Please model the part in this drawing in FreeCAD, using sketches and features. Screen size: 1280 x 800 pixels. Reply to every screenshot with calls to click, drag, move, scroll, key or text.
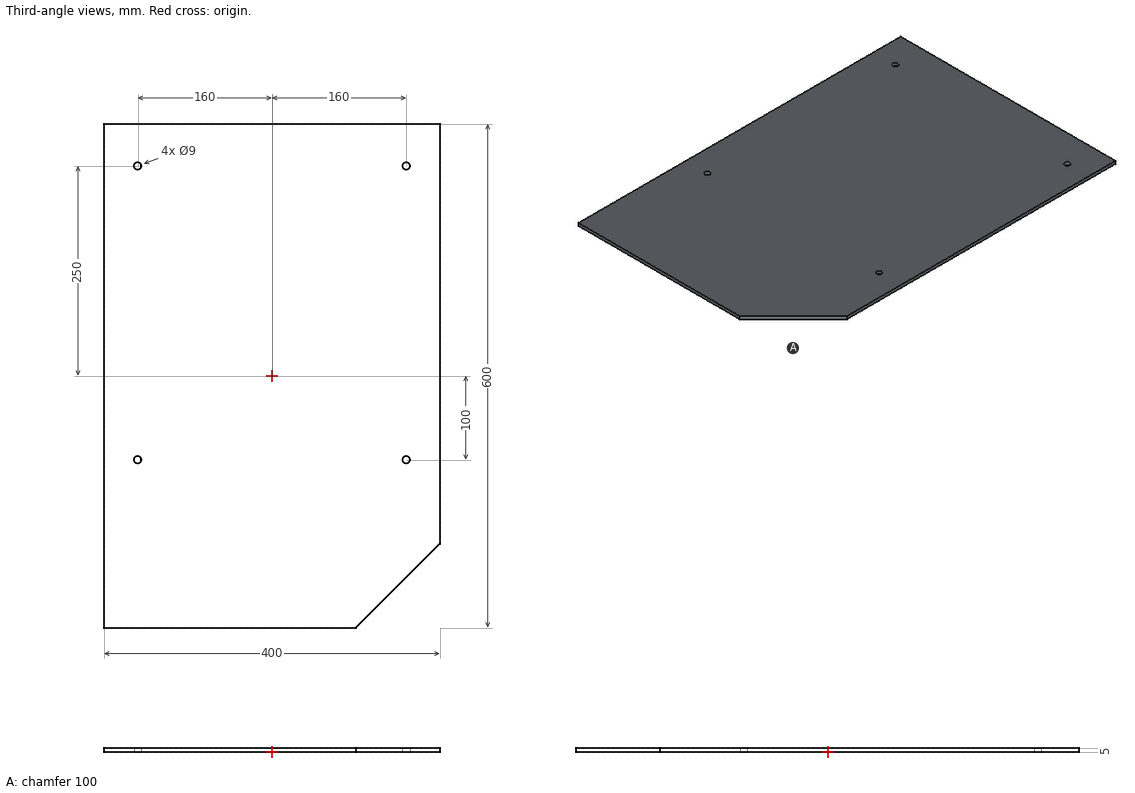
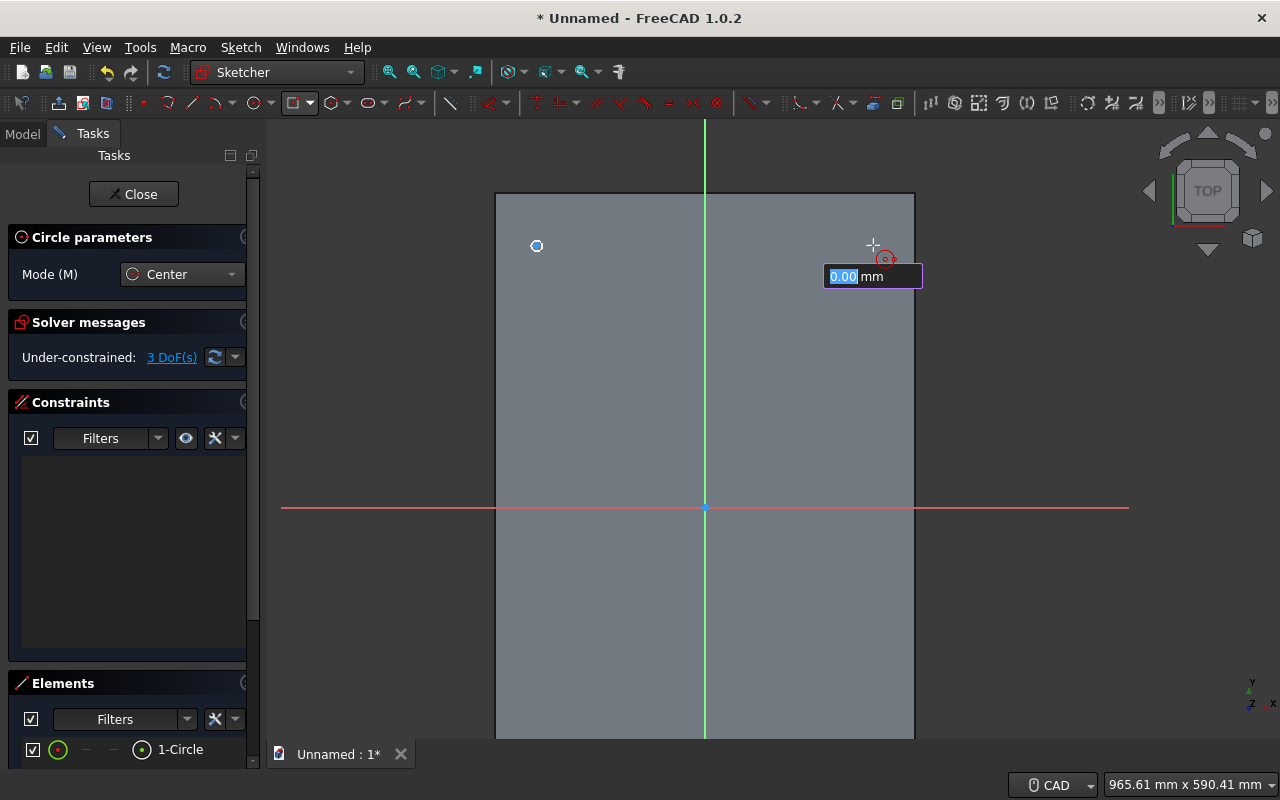
scroll(877, 242, up, 7)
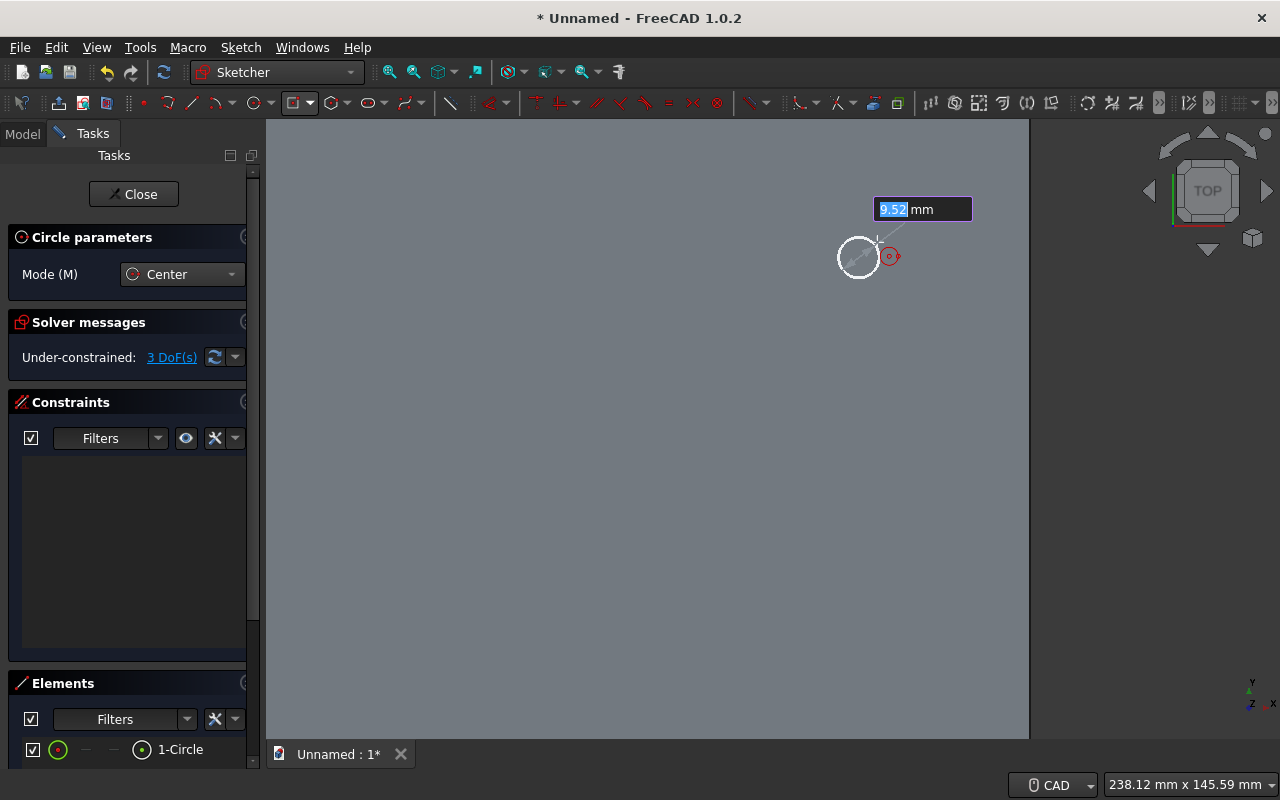
click(873, 241)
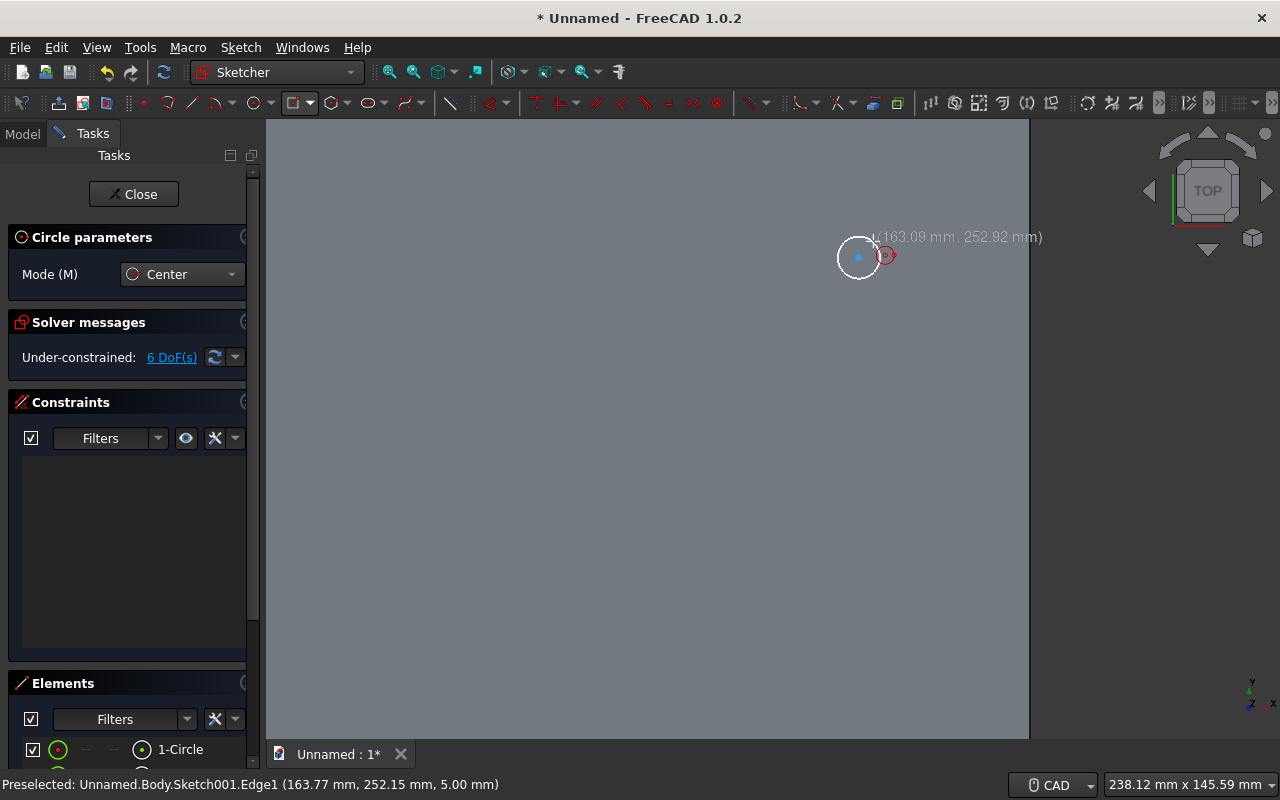
scroll(877, 242, down, 7)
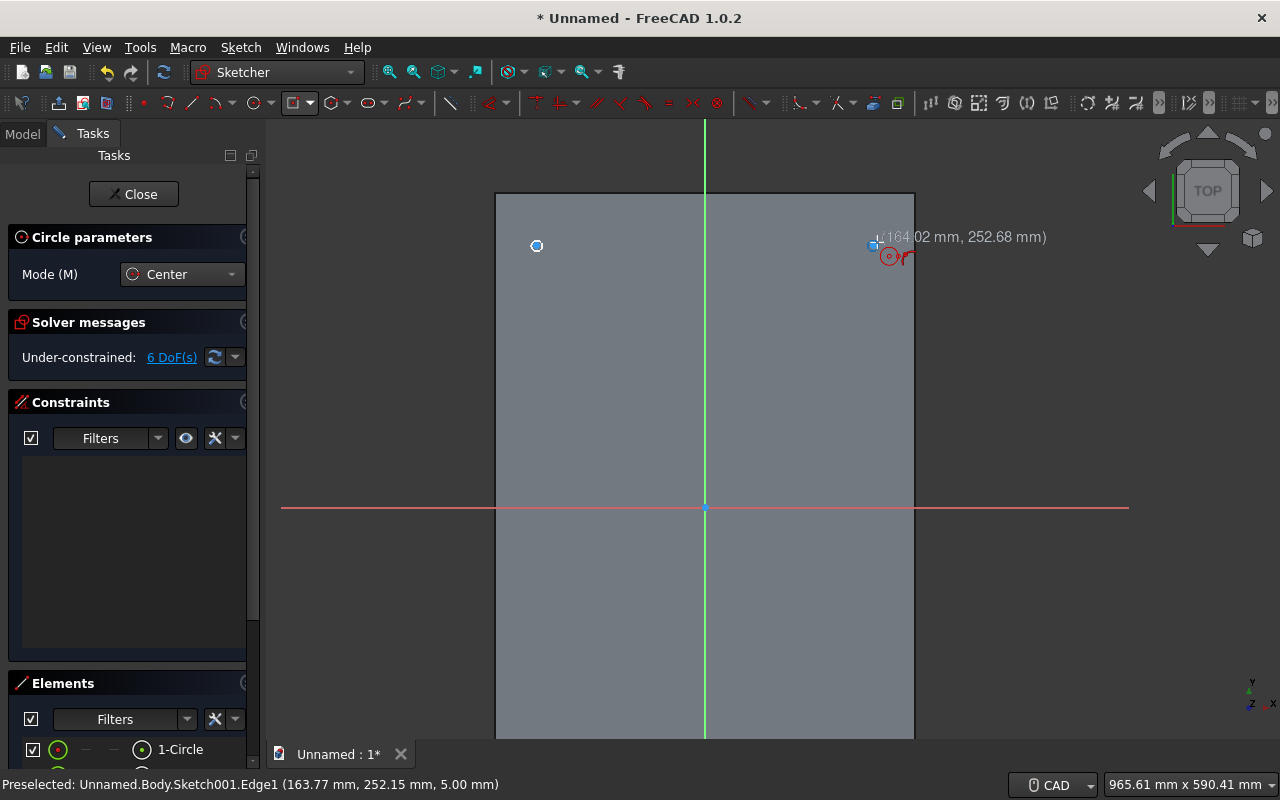
scroll(873, 613, up, 8)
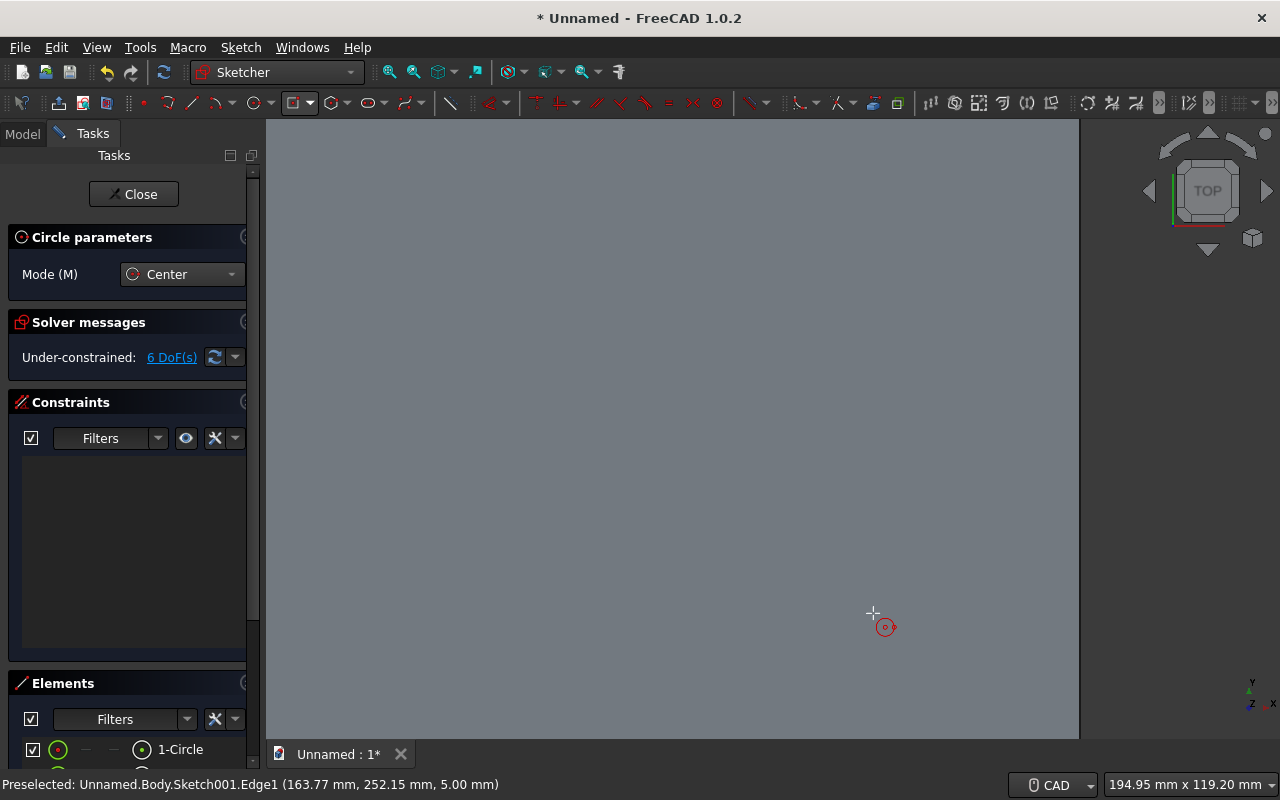
scroll(873, 614, down, 8)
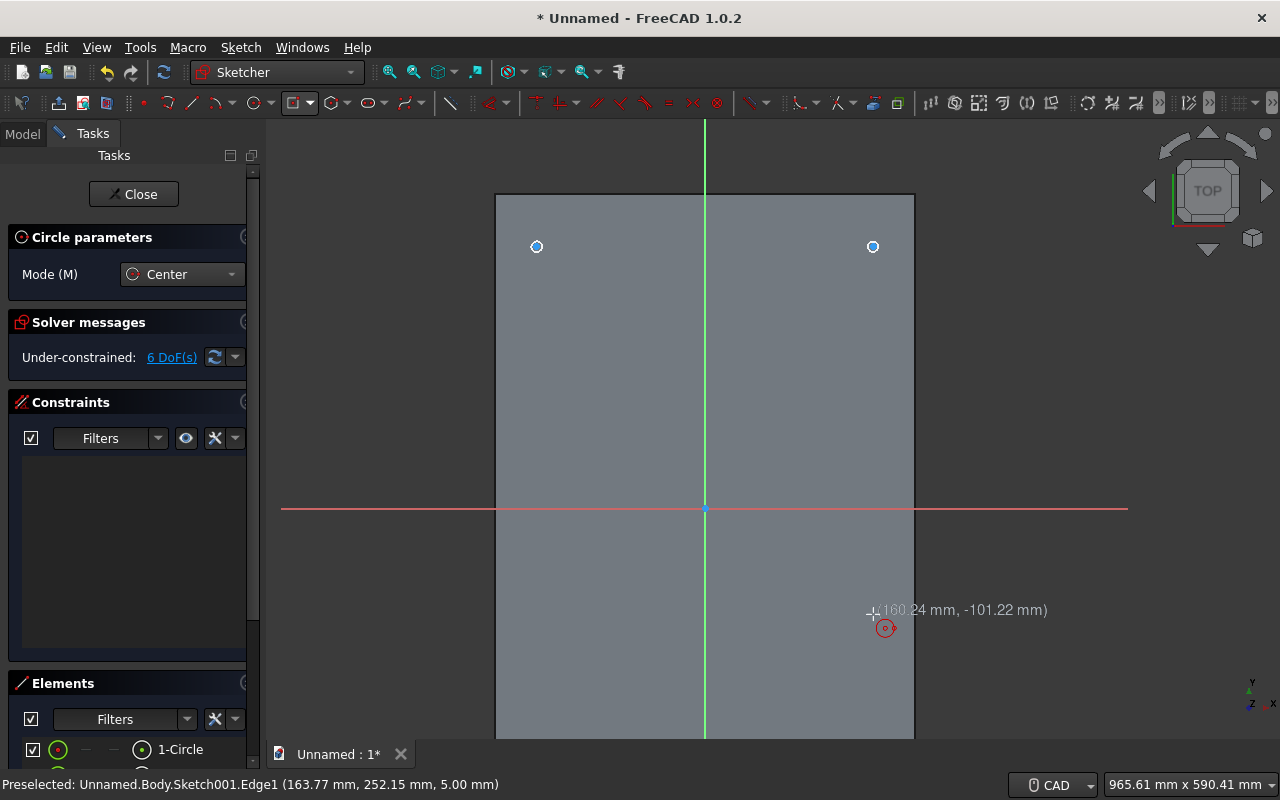
click(873, 614)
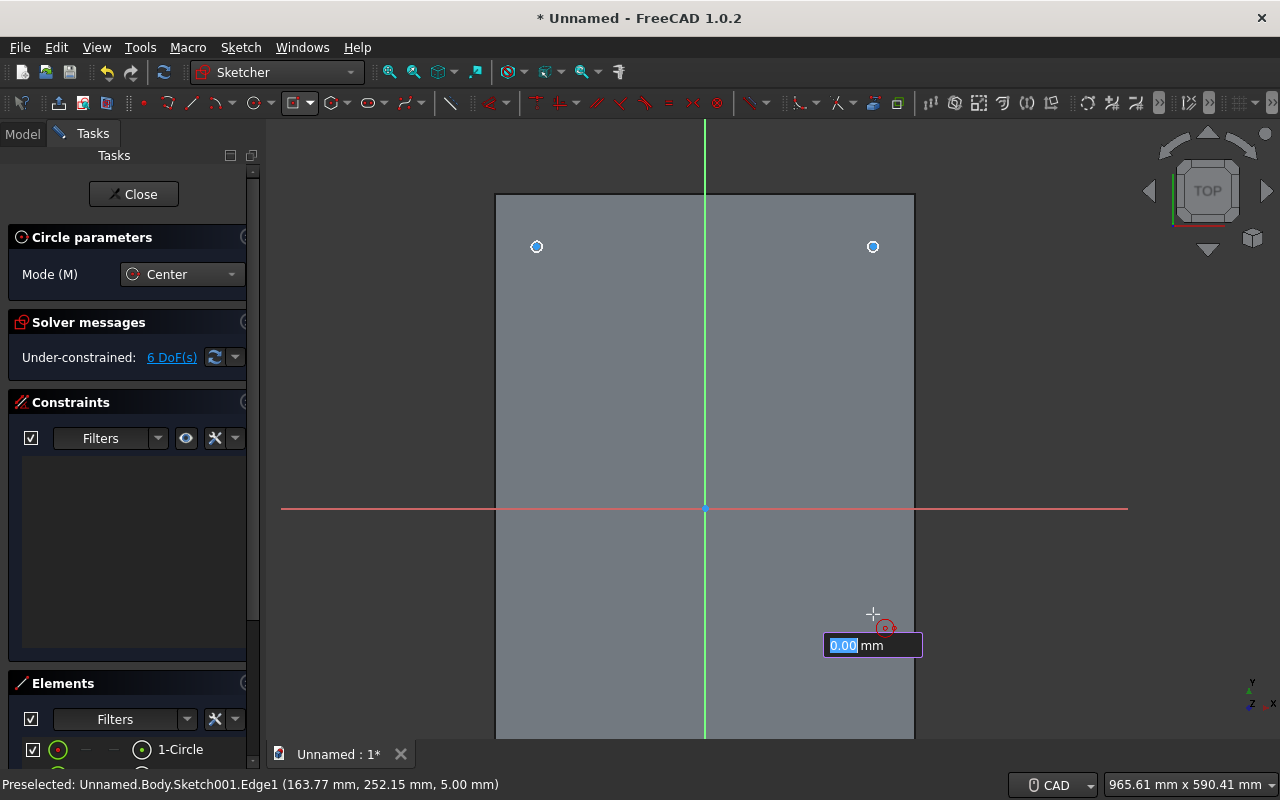
scroll(877, 610, up, 7)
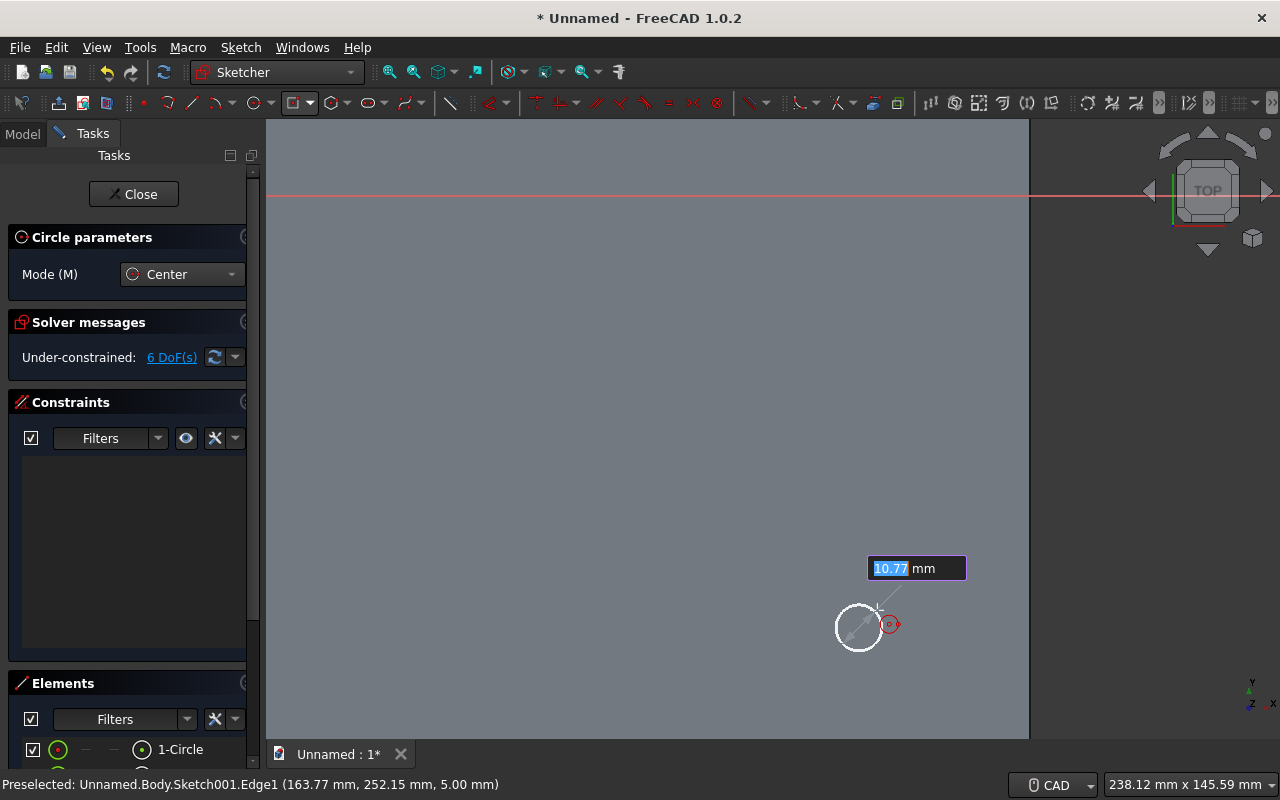
click(873, 608)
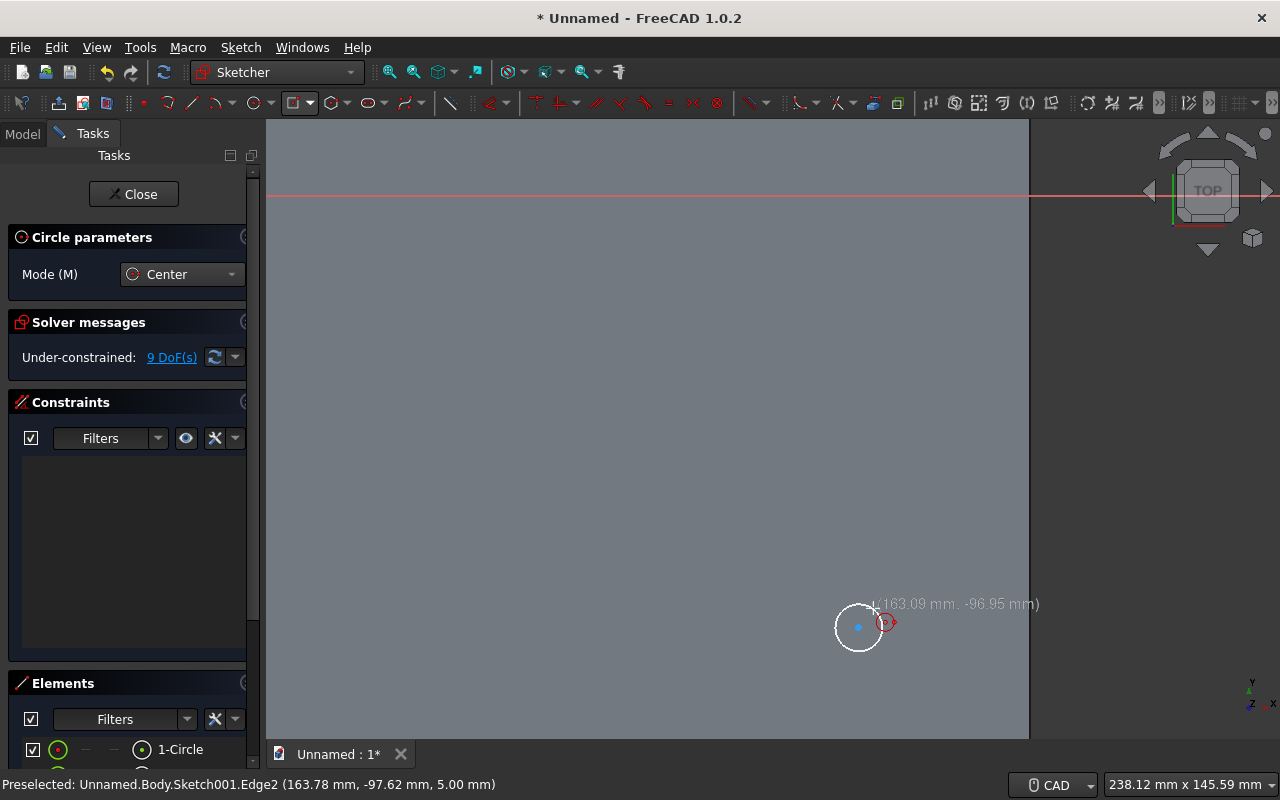
scroll(877, 610, down, 7)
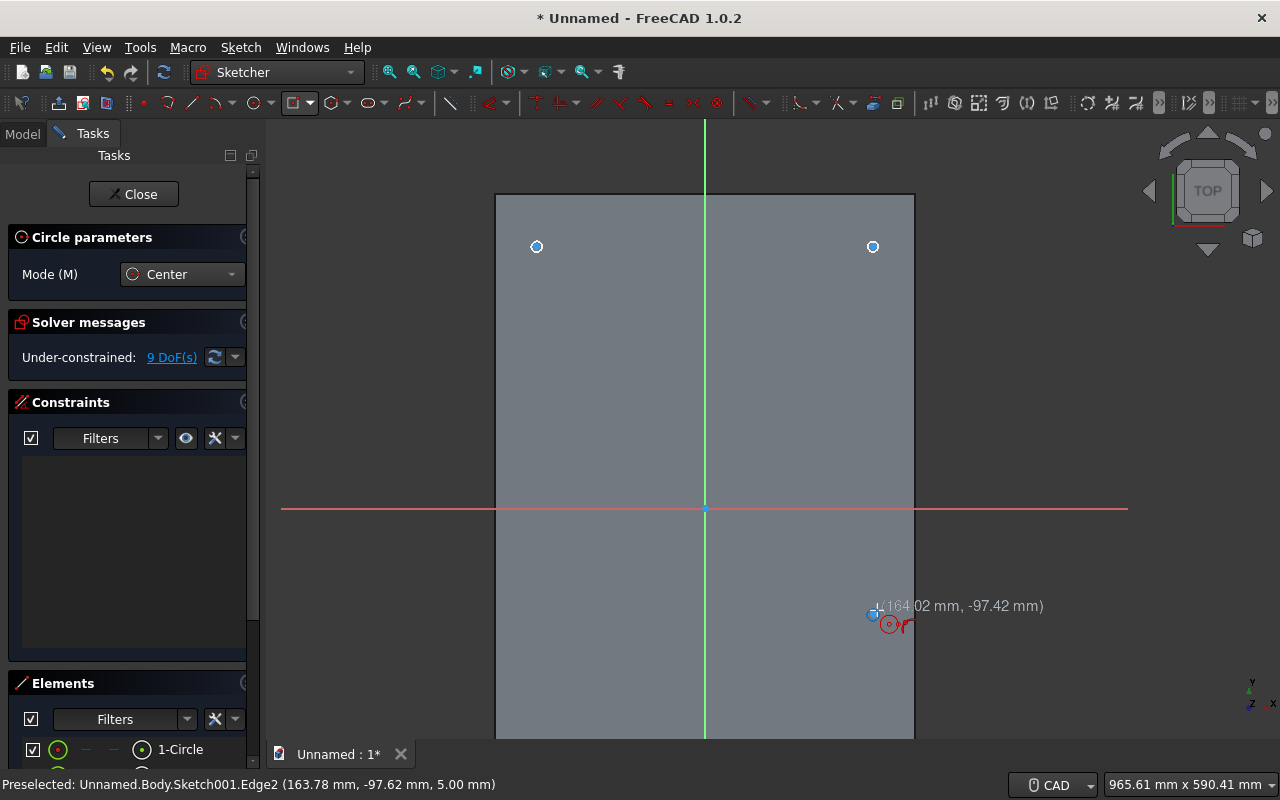
scroll(537, 614, up, 8)